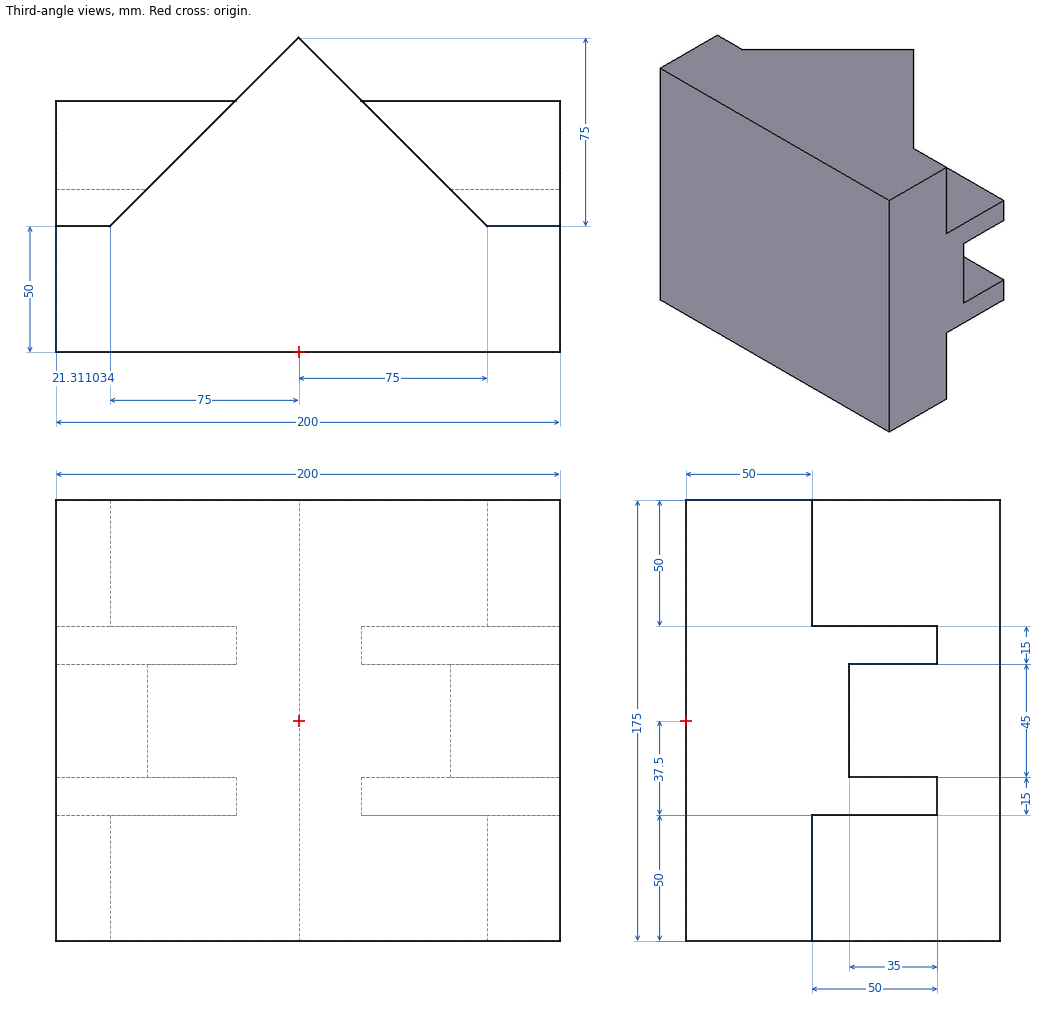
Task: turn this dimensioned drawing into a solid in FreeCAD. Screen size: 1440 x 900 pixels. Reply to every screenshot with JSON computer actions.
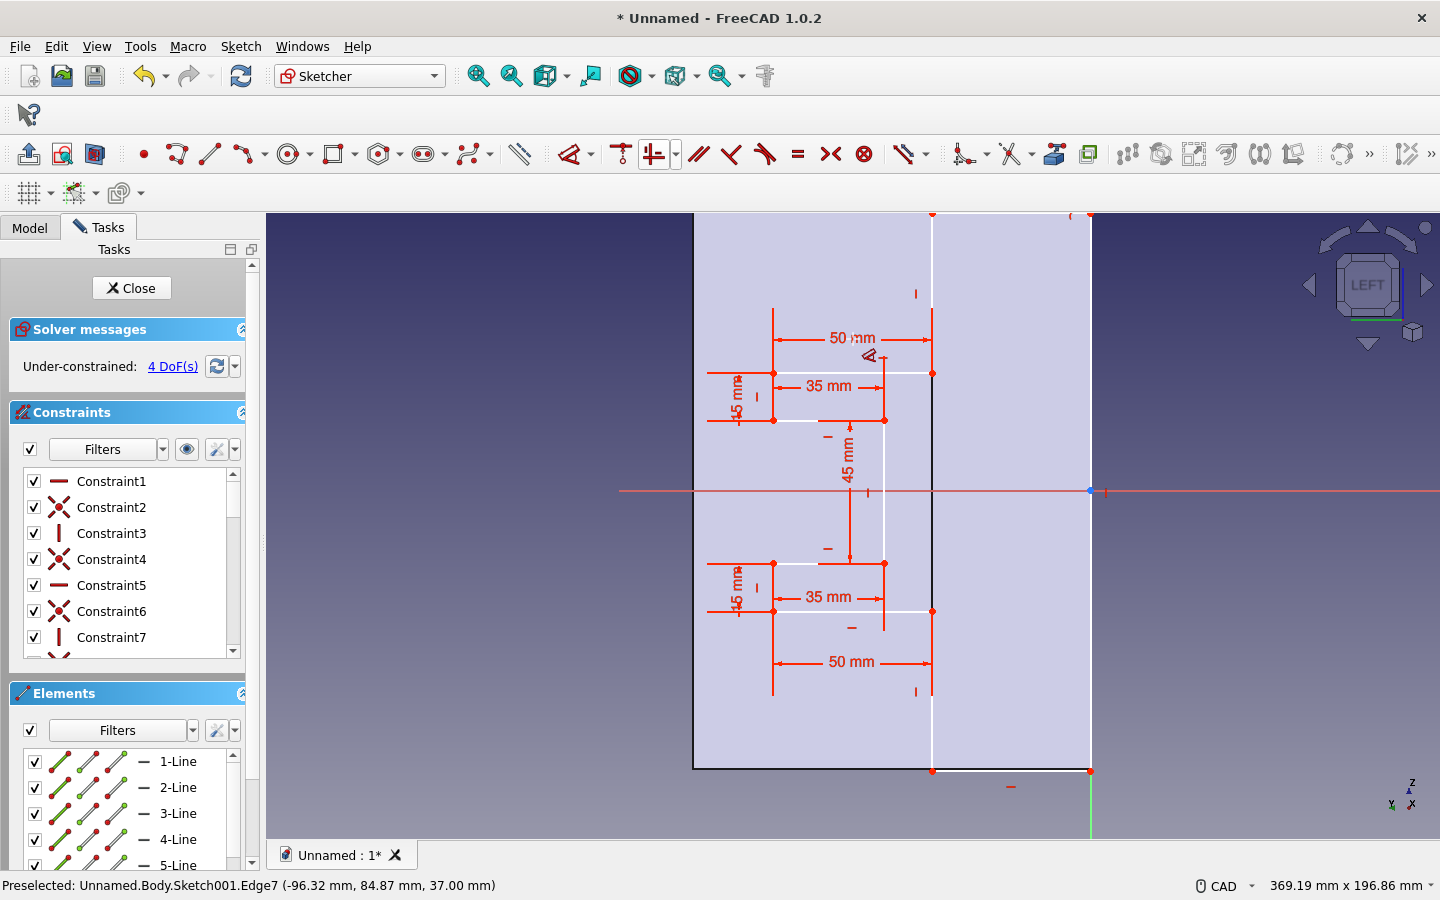
{"action": "left_click", "coordinate": [932, 325]}
{"action": "left_click", "coordinate": [966, 307]}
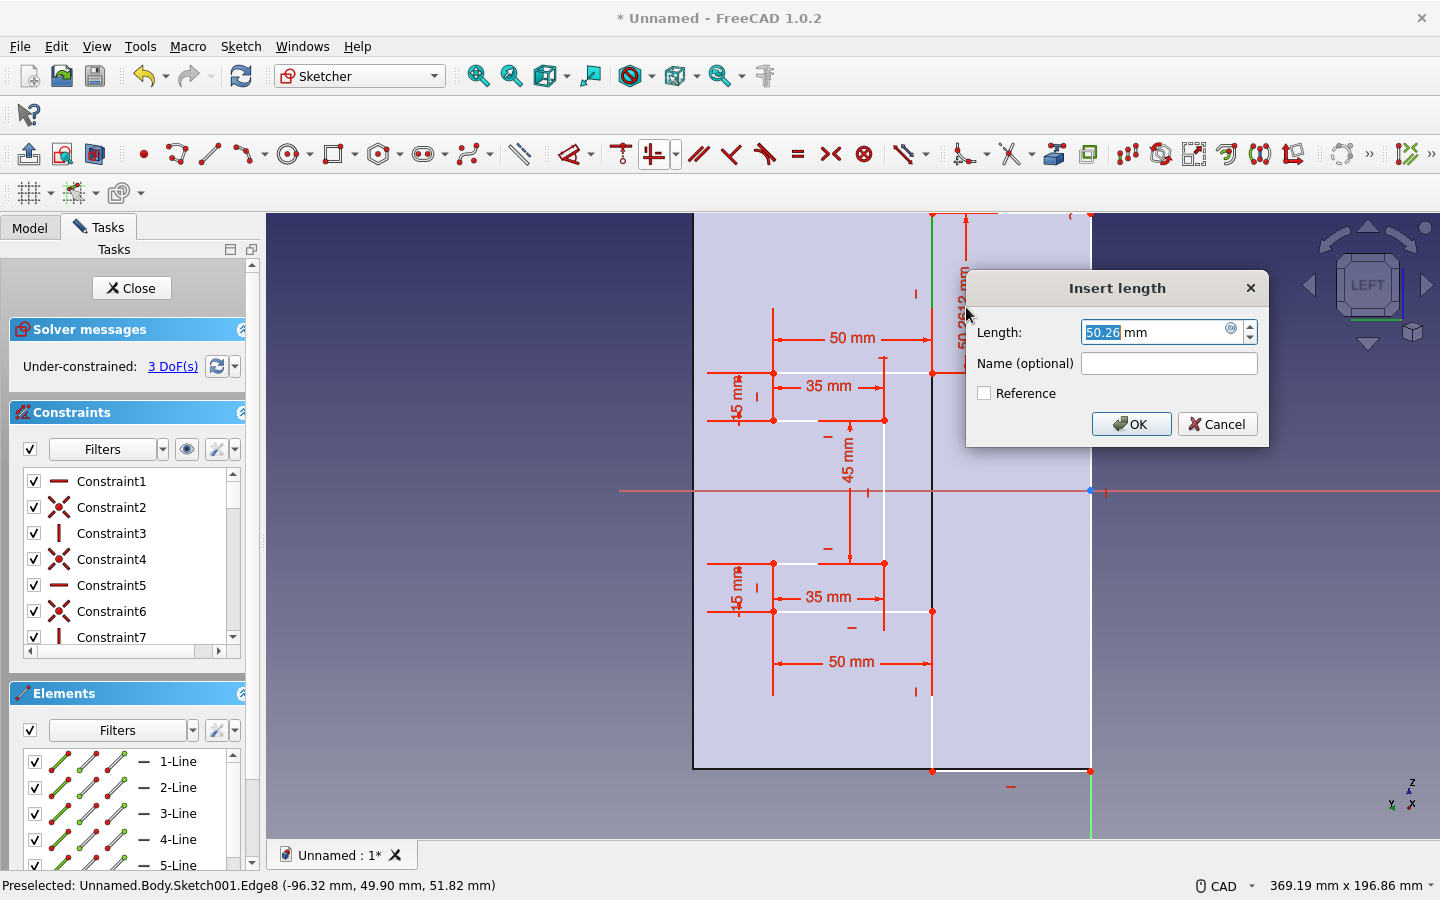
{"action": "type", "text": "50"}
{"action": "key", "text": "Return"}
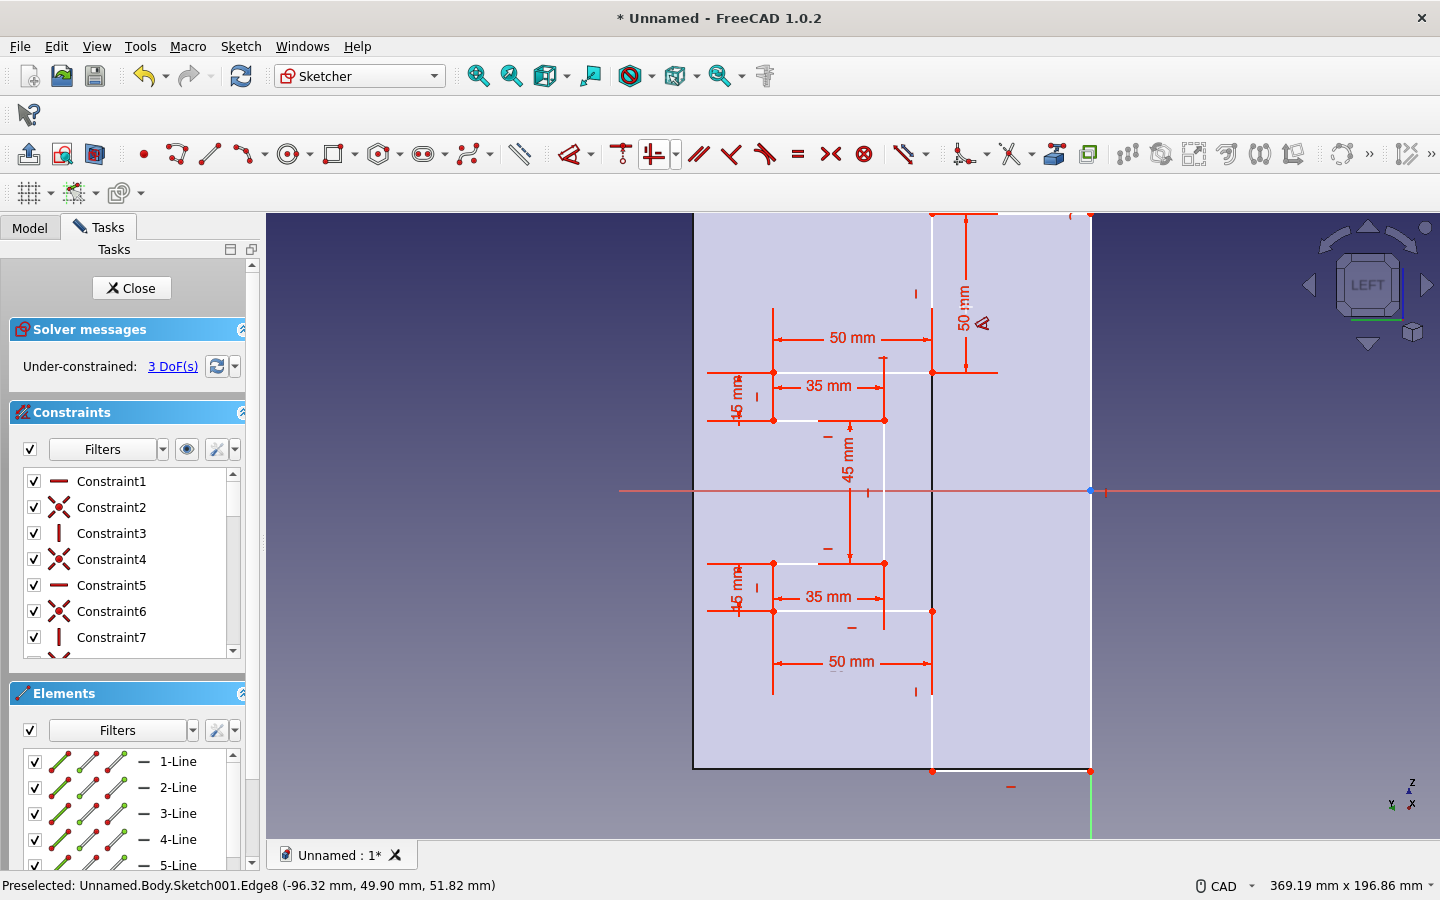
{"action": "scroll", "coordinate": [485, 598], "scroll_direction": "down", "scroll_amount": 2}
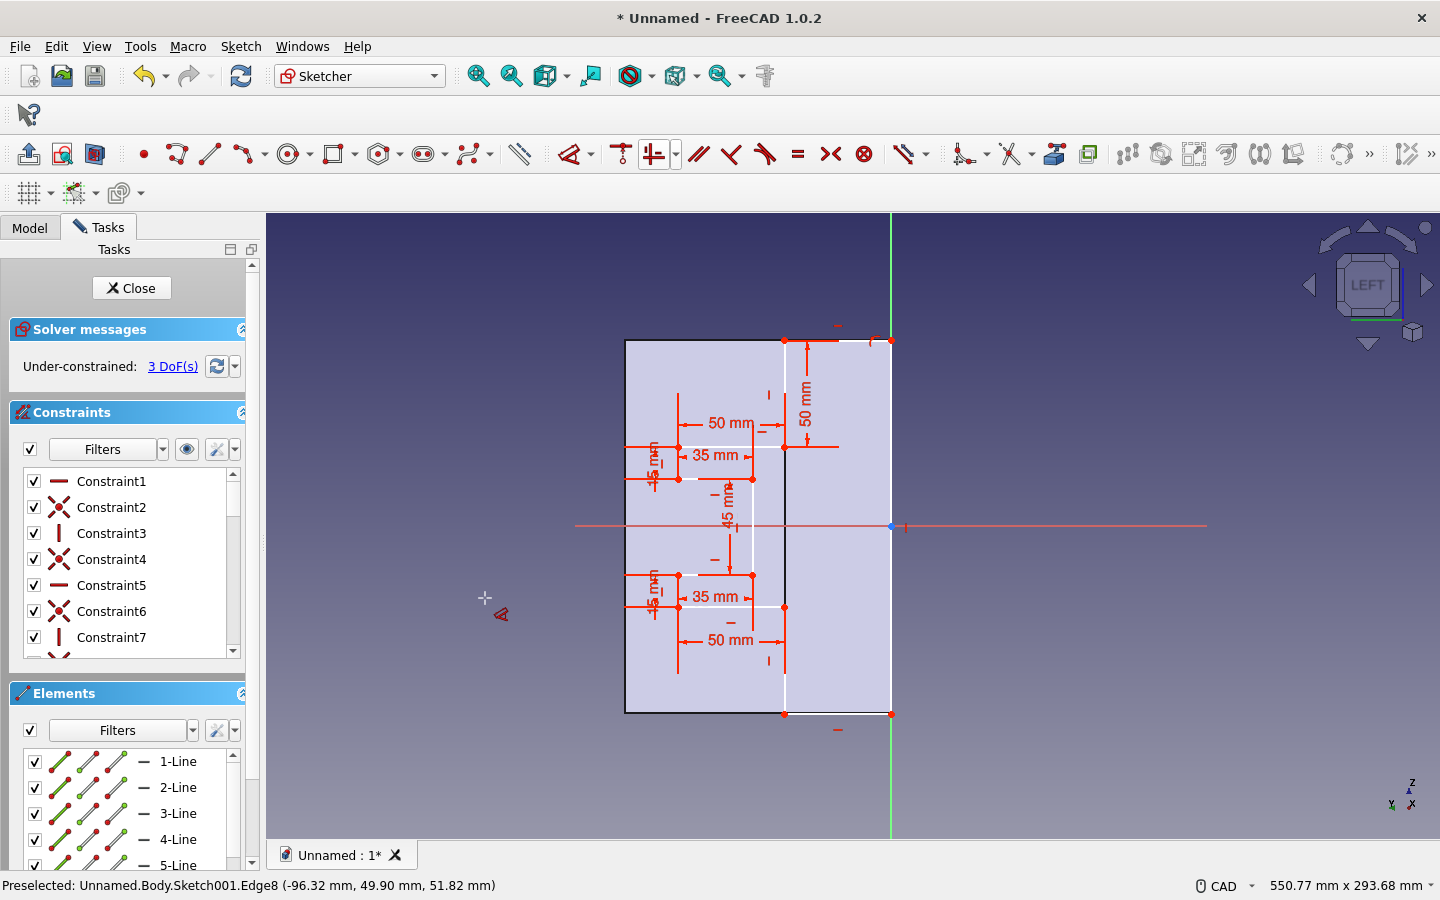
{"action": "left_click", "coordinate": [817, 341]}
{"action": "left_click", "coordinate": [838, 307]}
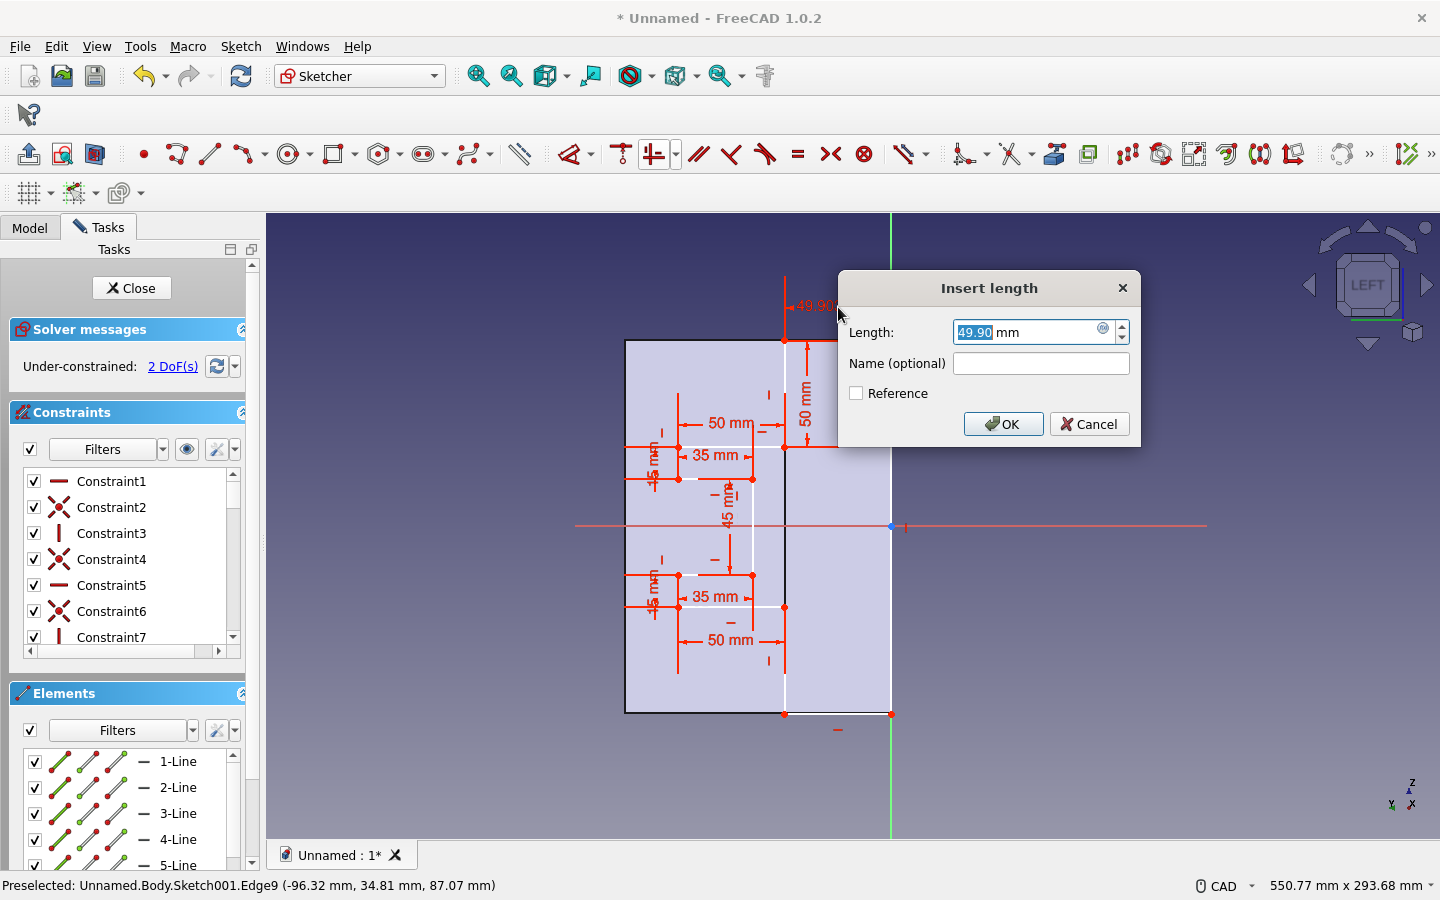
{"action": "type", "text": "50"}
{"action": "key", "text": "Return"}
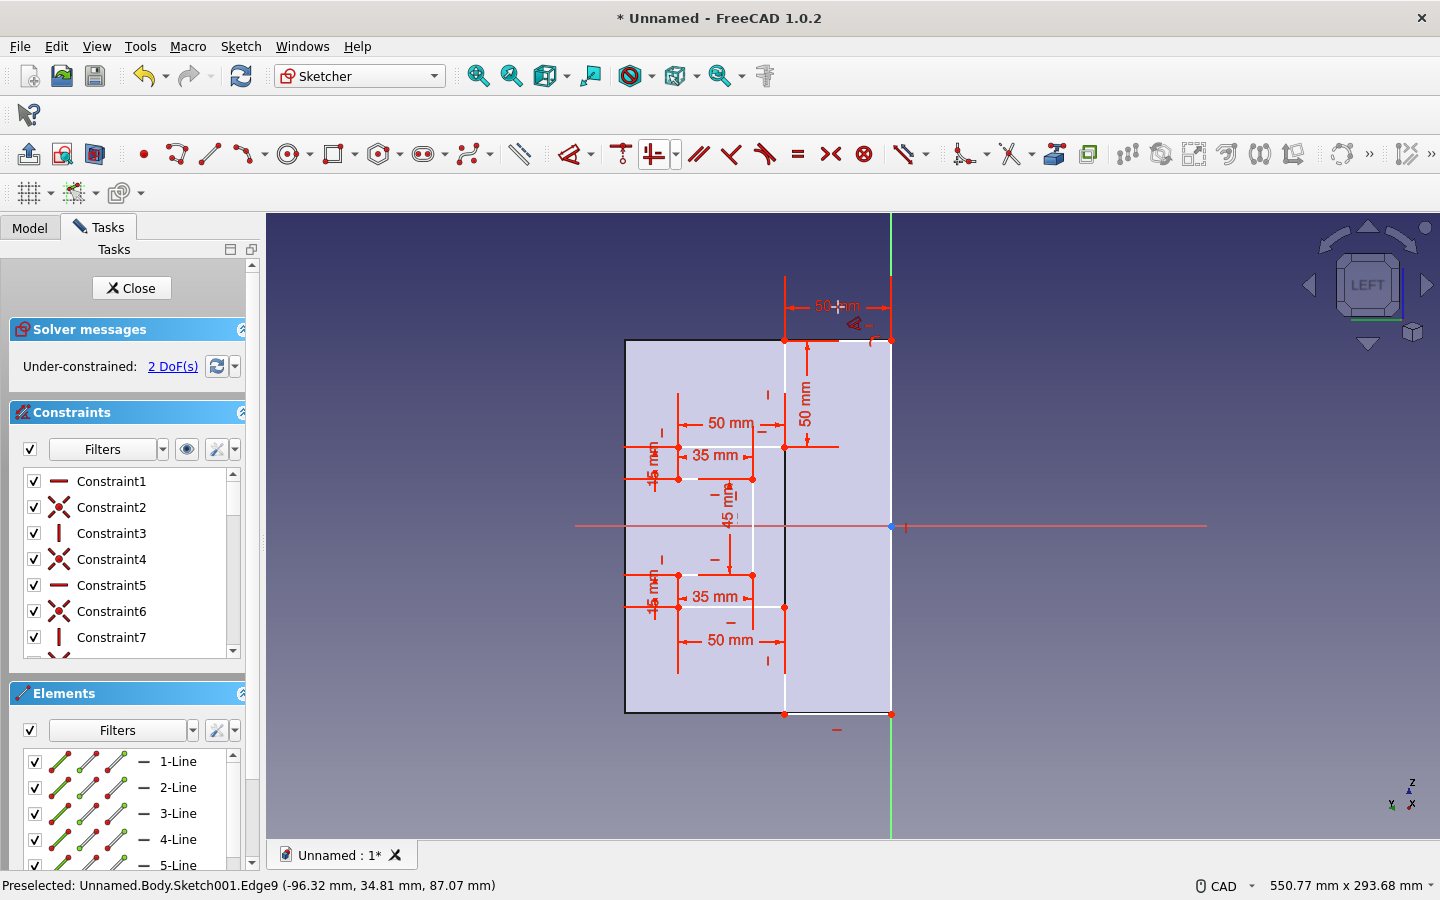
{"action": "left_click", "coordinate": [785, 682]}
{"action": "left_click", "coordinate": [819, 661]}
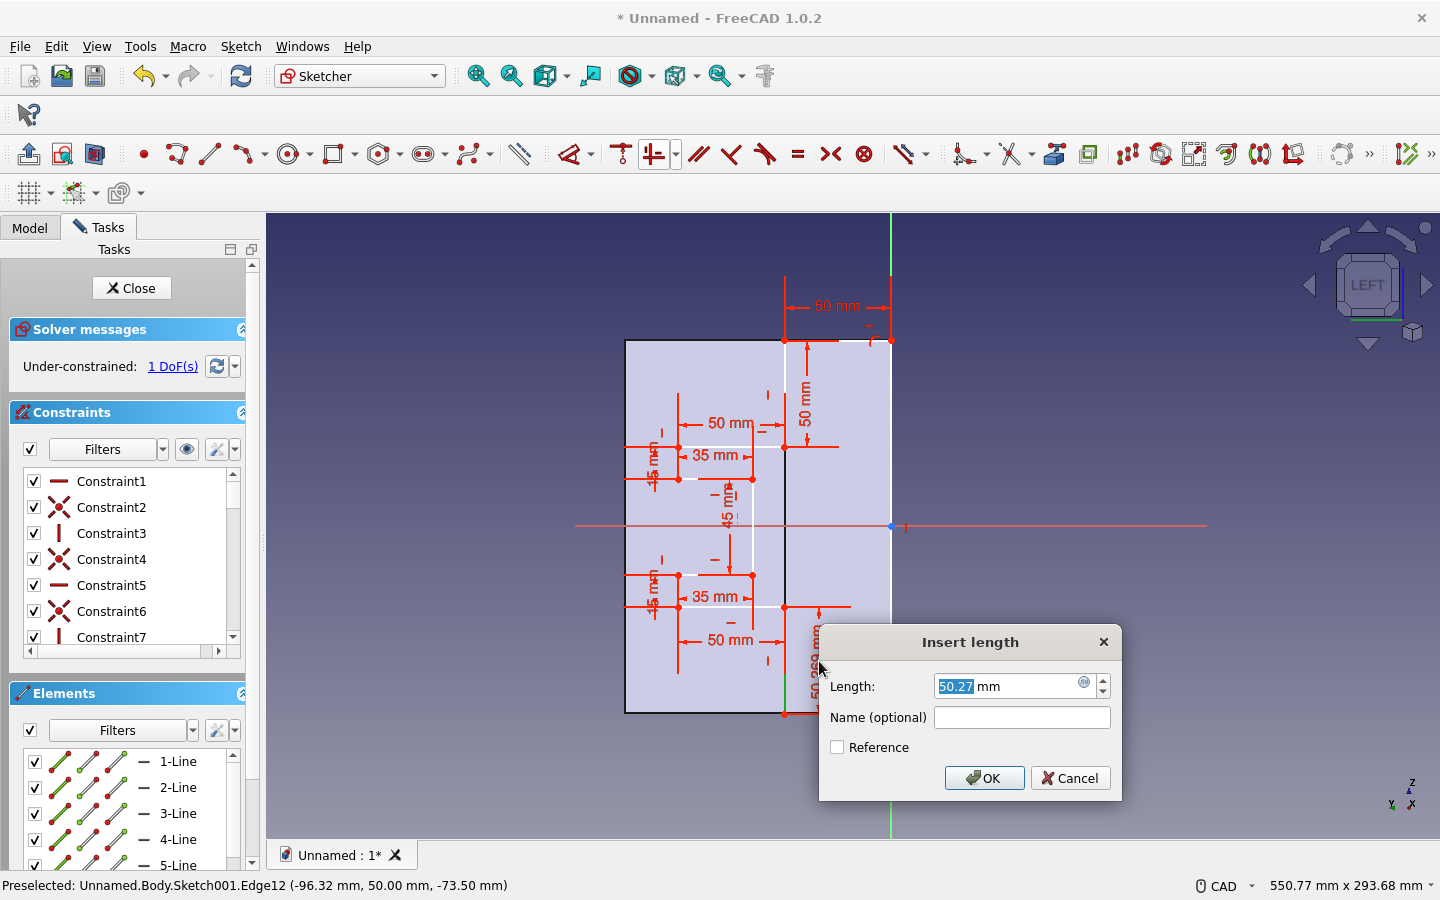
{"action": "type", "text": "50"}
{"action": "key", "text": "Return"}